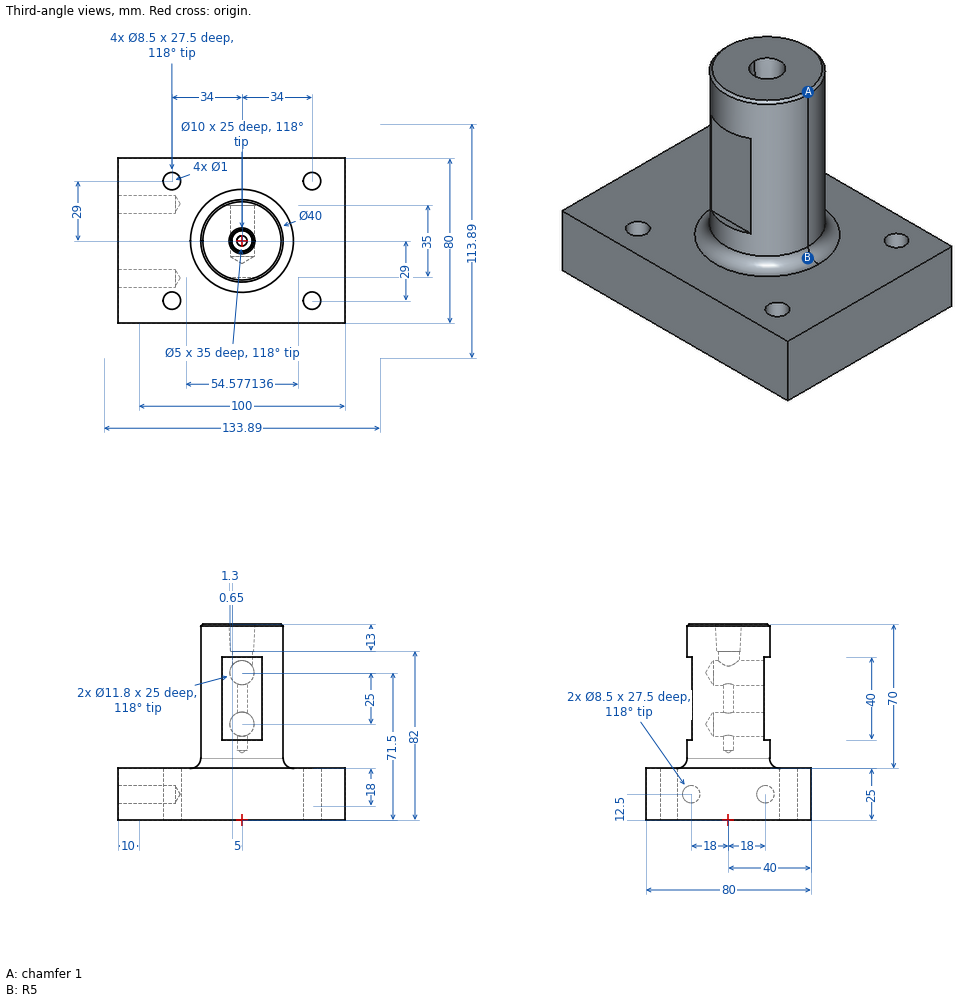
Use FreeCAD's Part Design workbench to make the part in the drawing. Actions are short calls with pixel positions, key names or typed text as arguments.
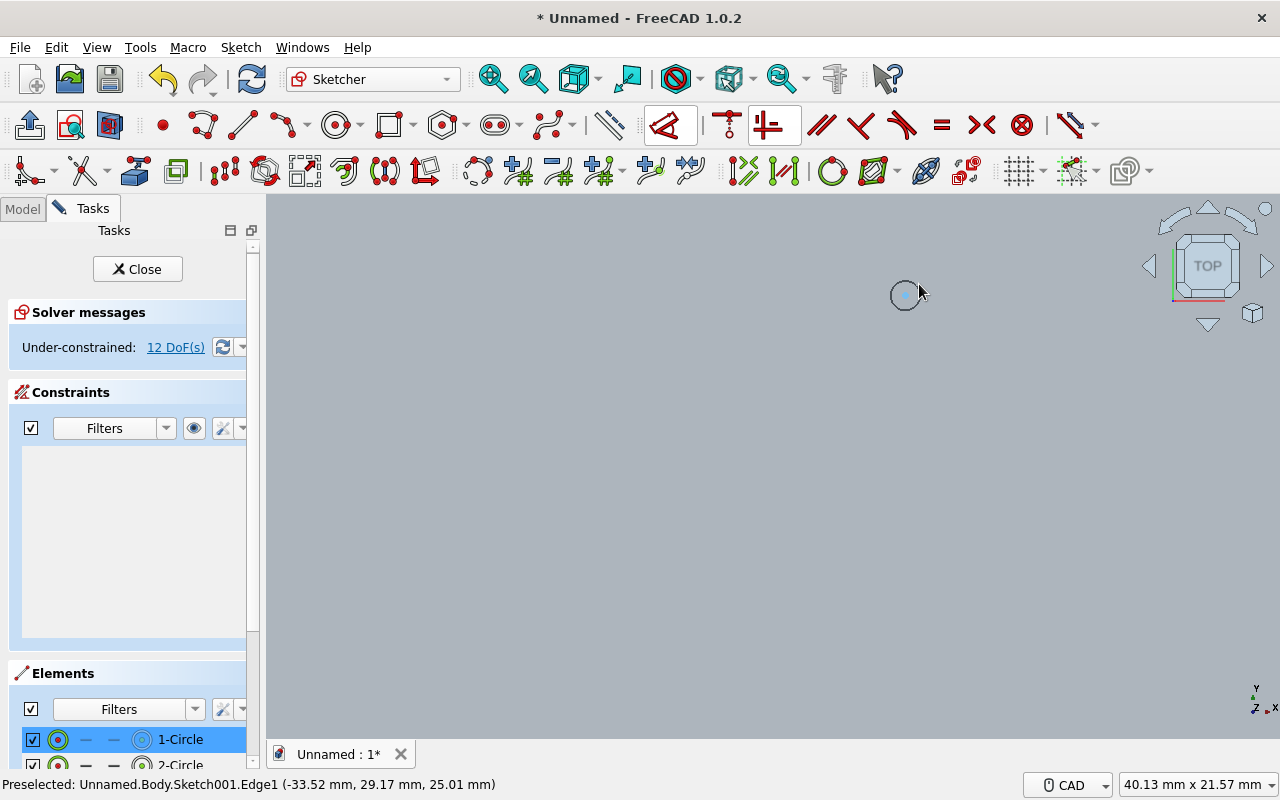
click(916, 285)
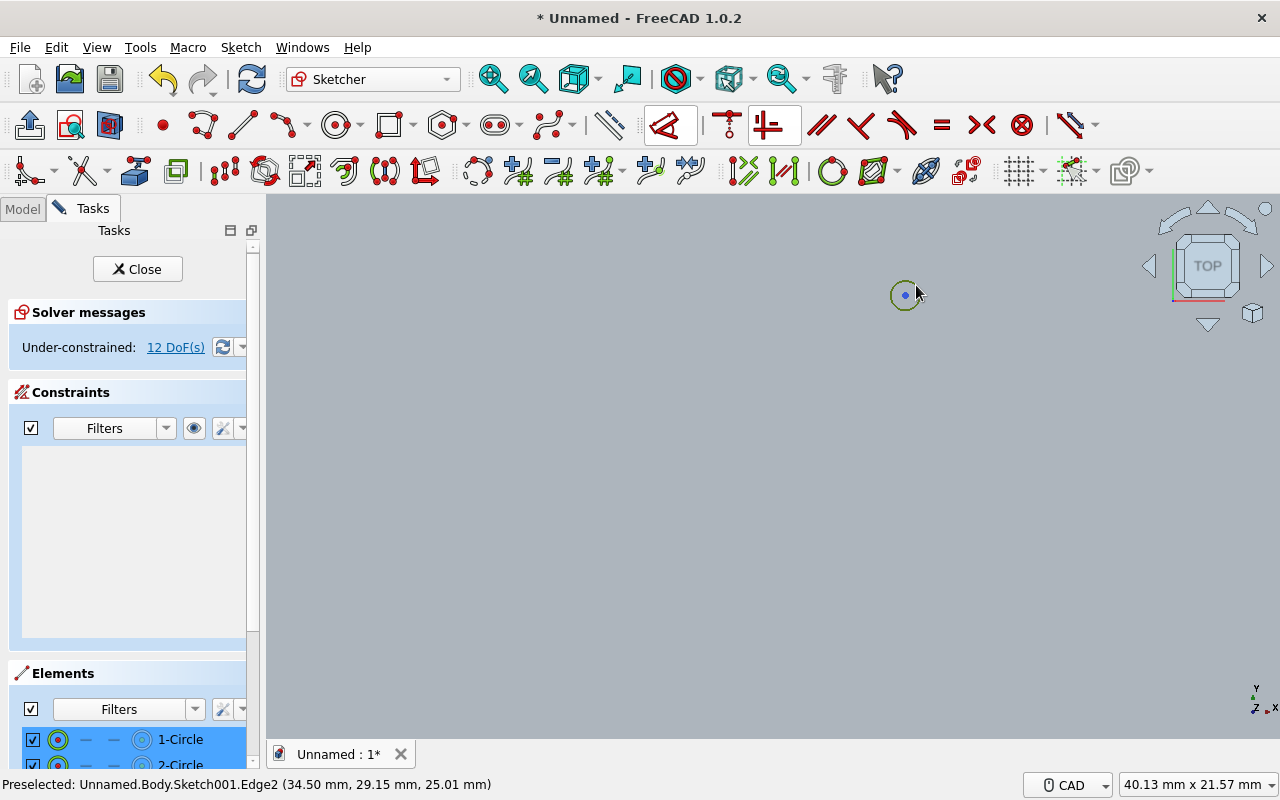
scroll(920, 284, down, 7)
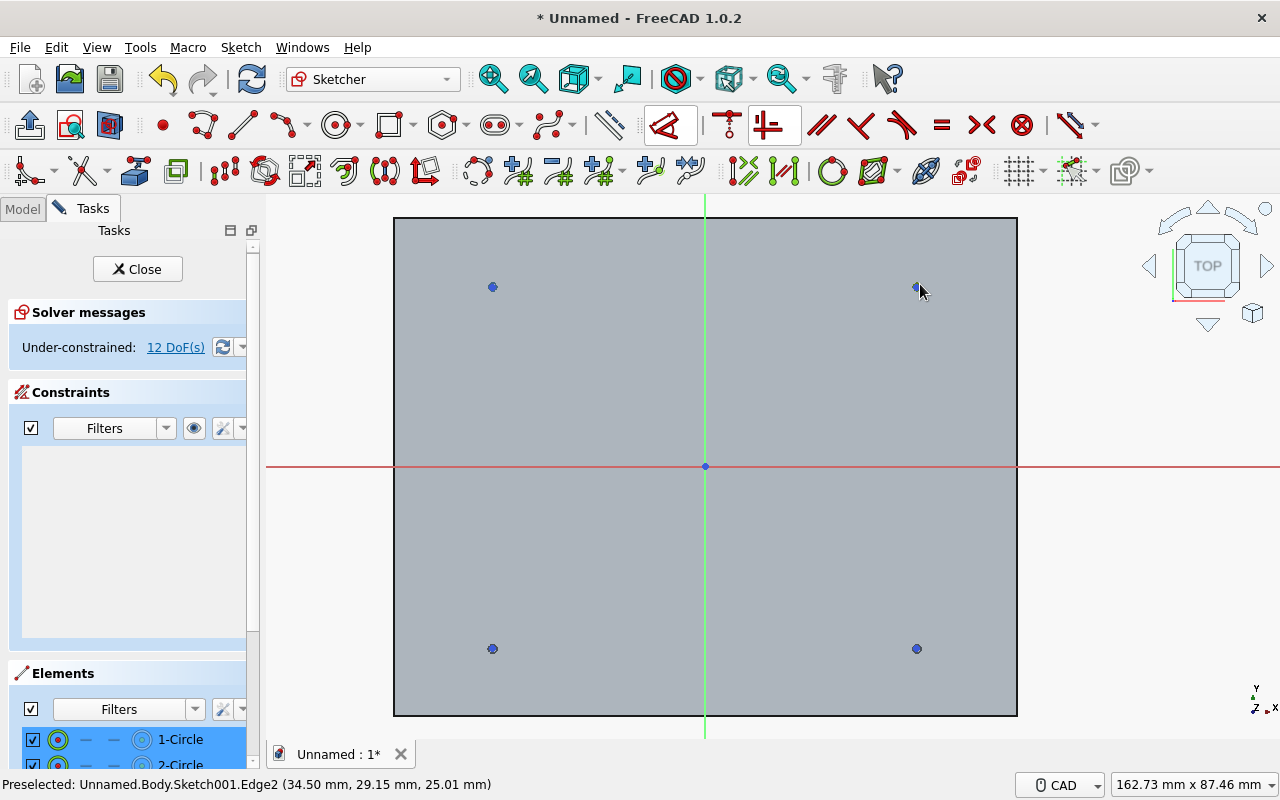
scroll(920, 646, up, 7)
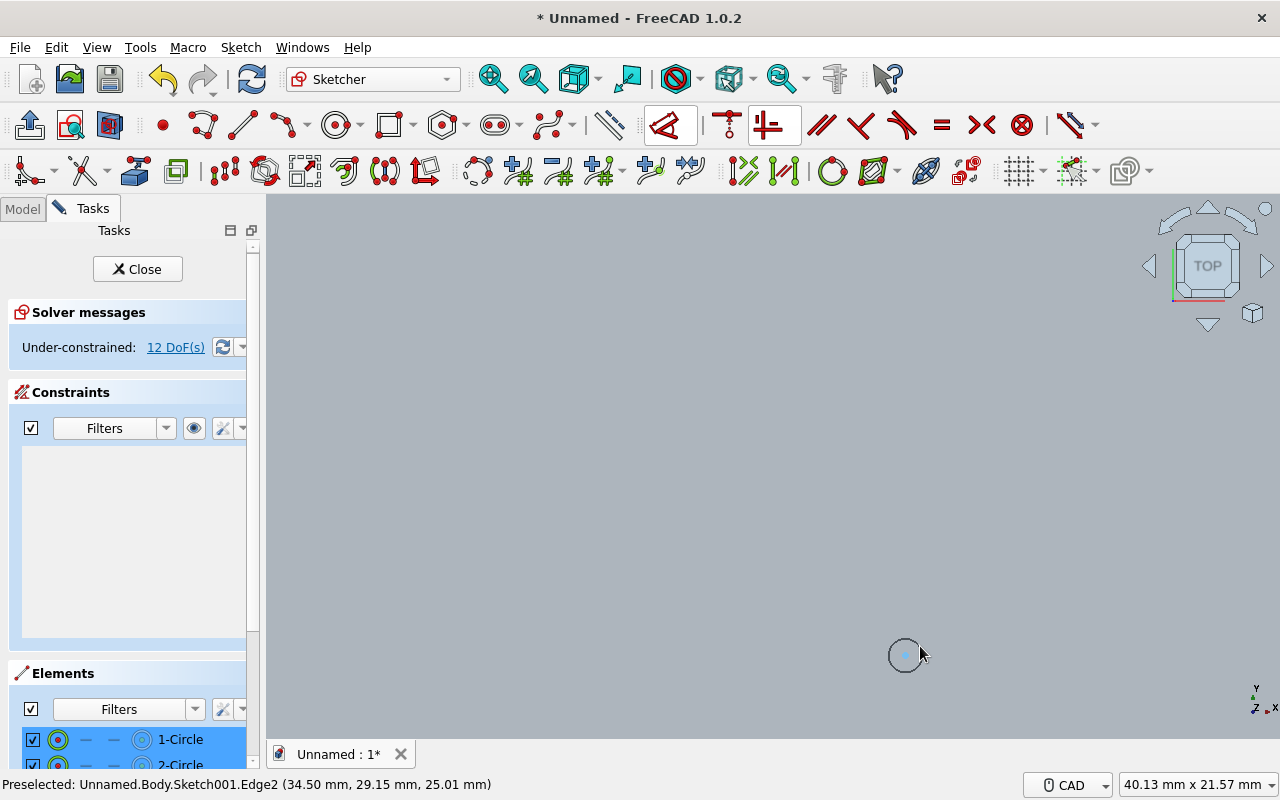
click(917, 644)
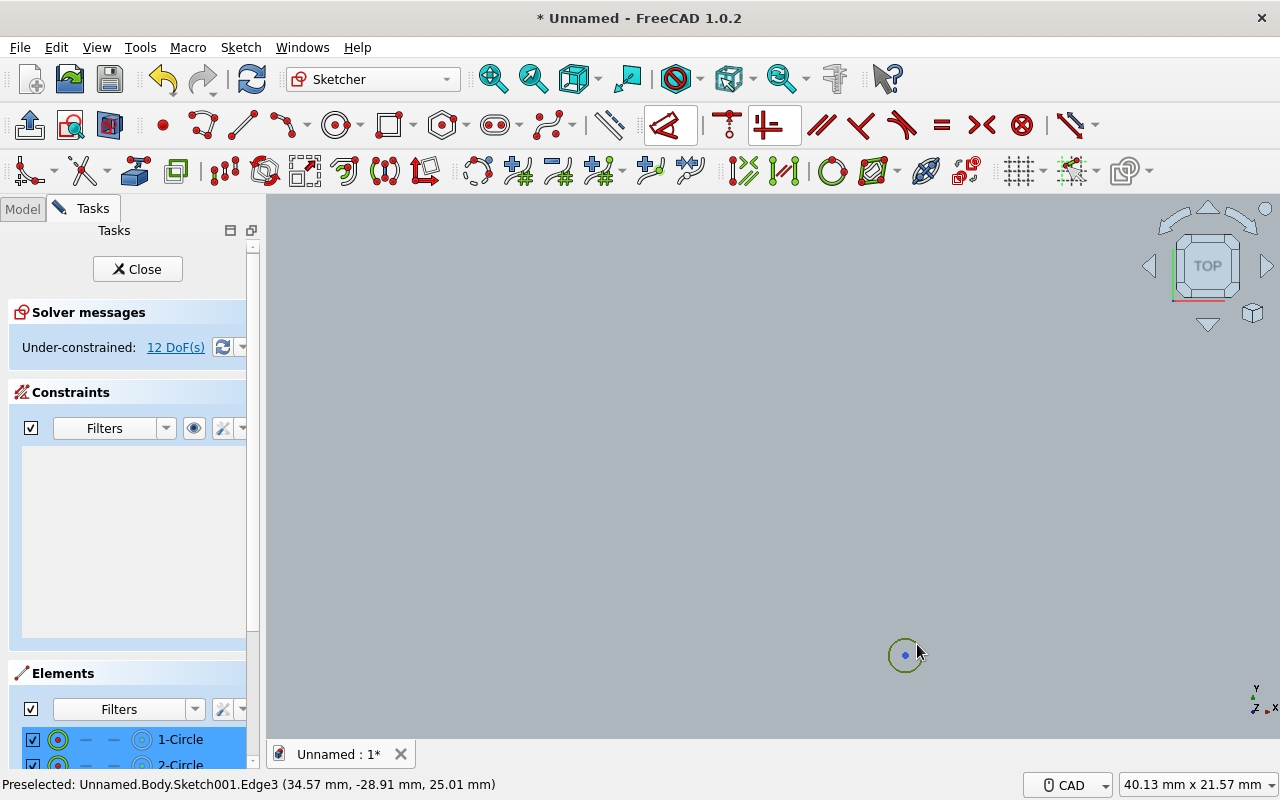
scroll(920, 646, down, 7)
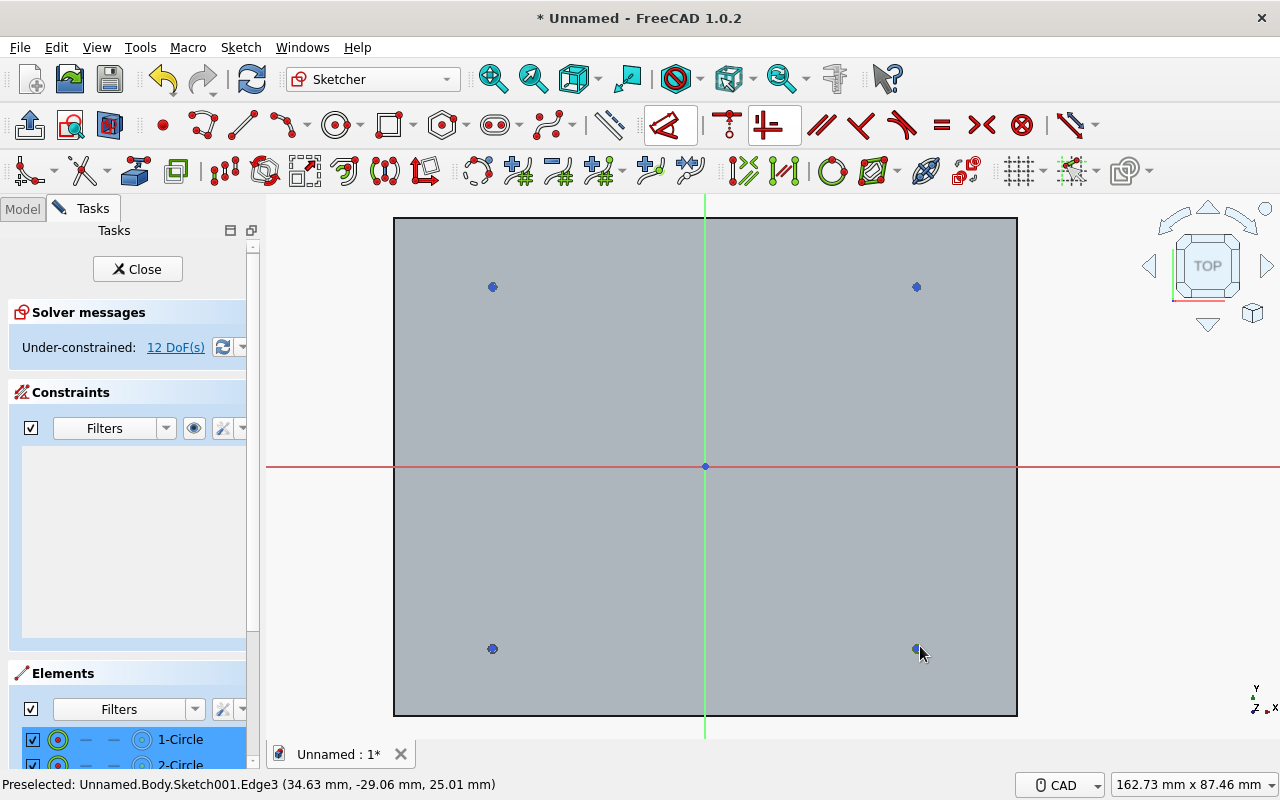
scroll(496, 646, up, 6)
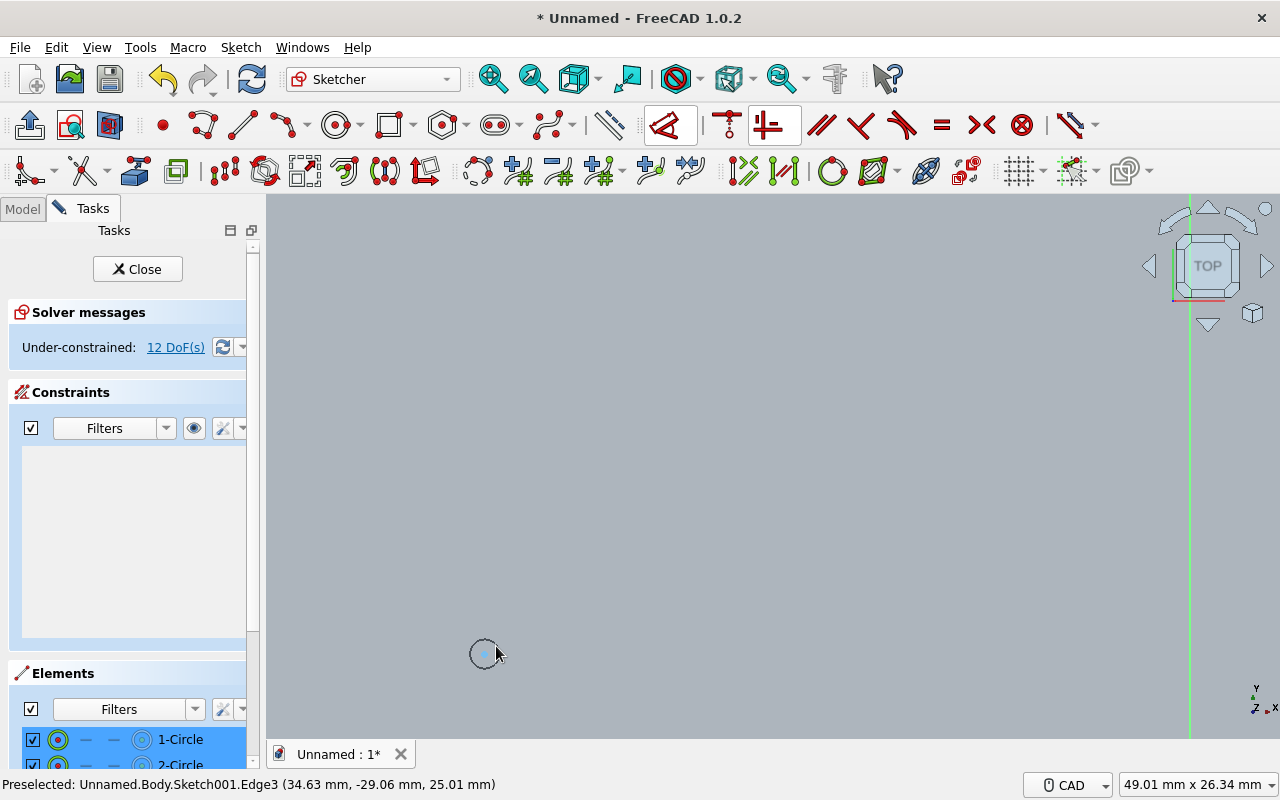
click(495, 644)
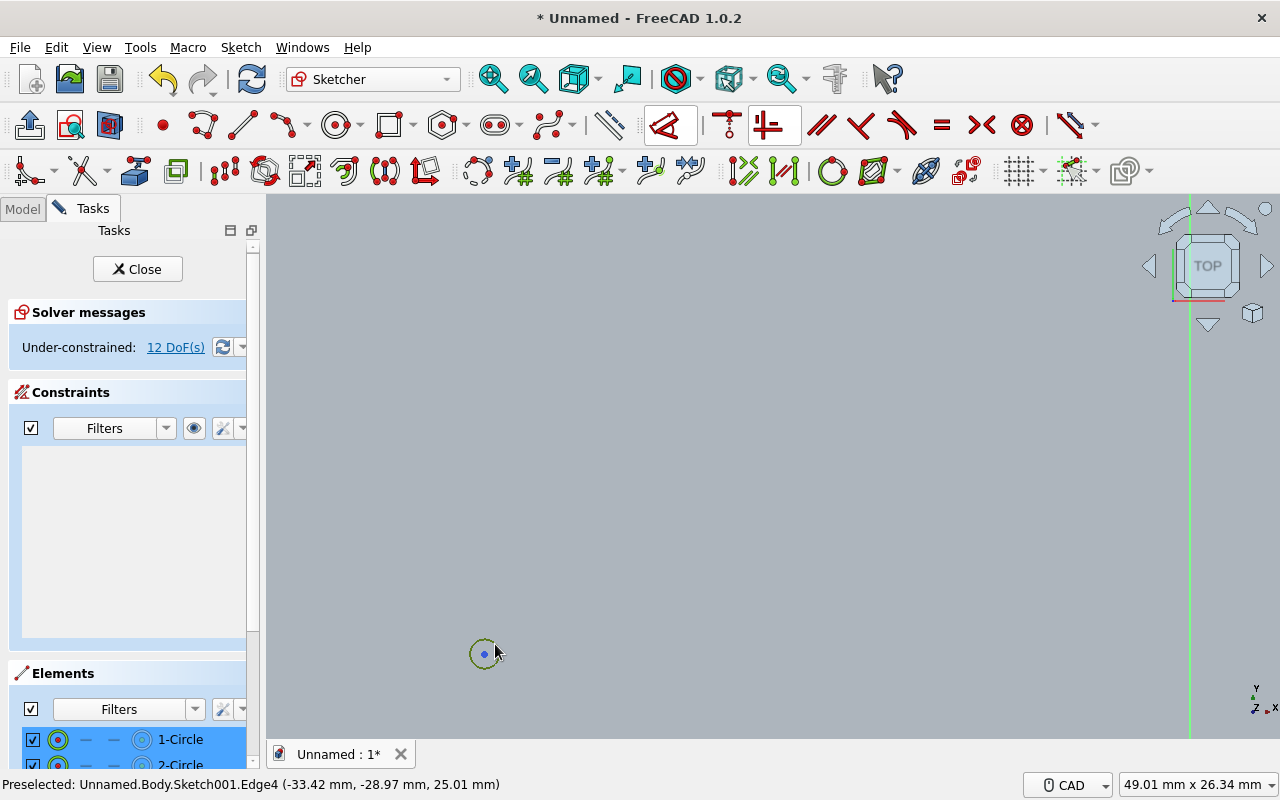
click(942, 126)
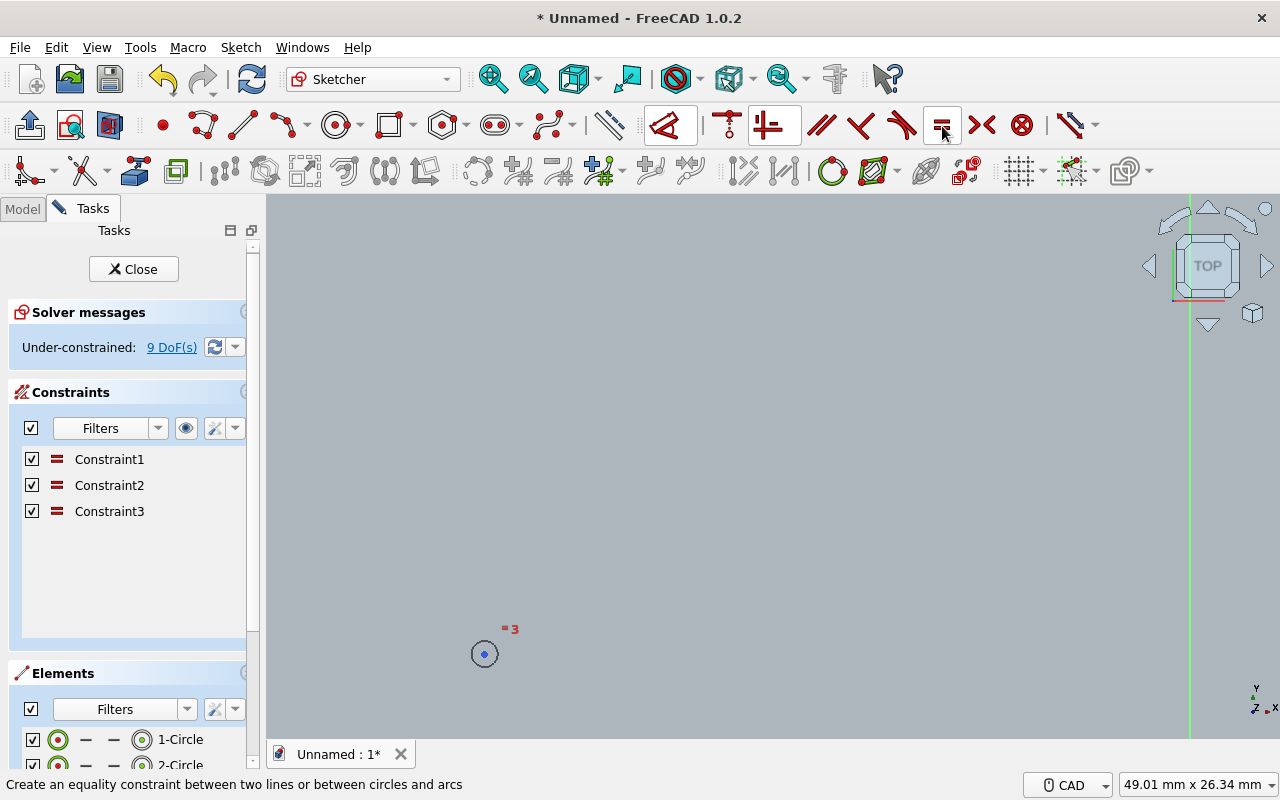
scroll(495, 646, down, 6)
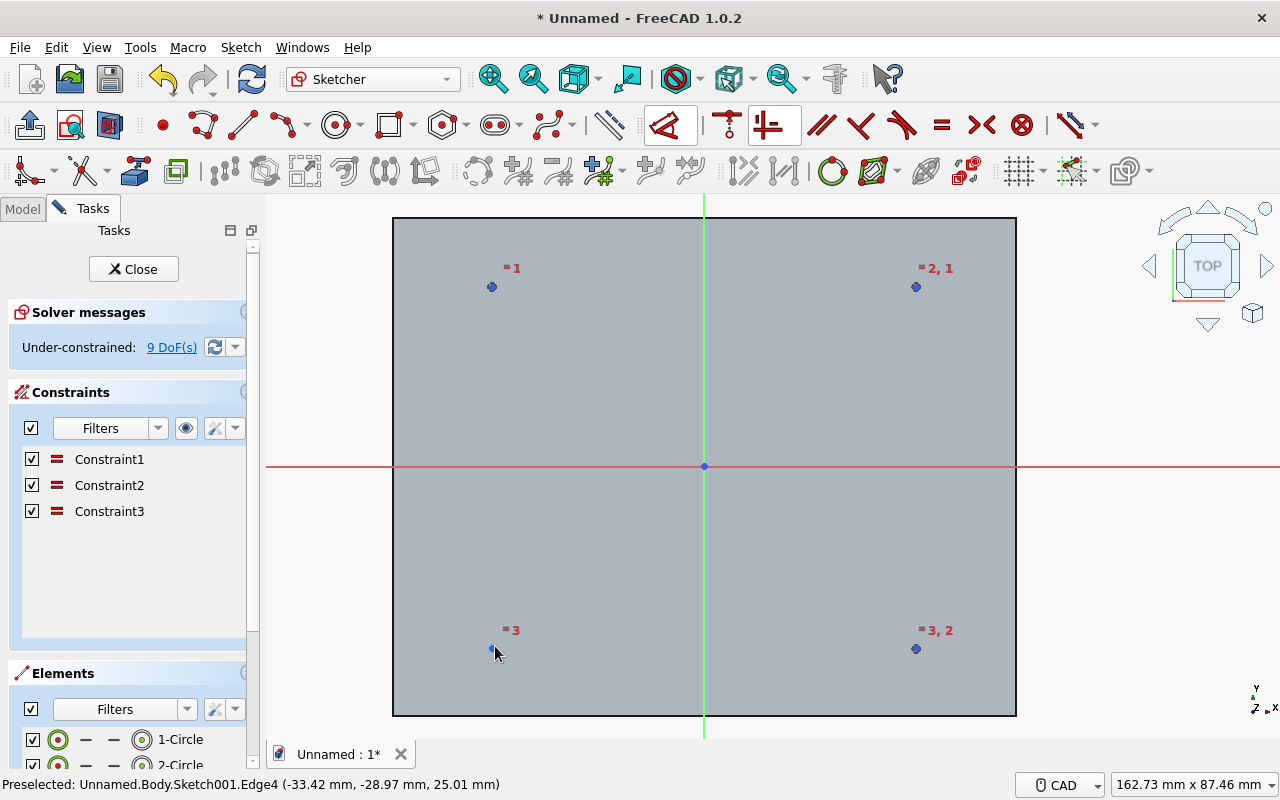
scroll(495, 284, up, 10)